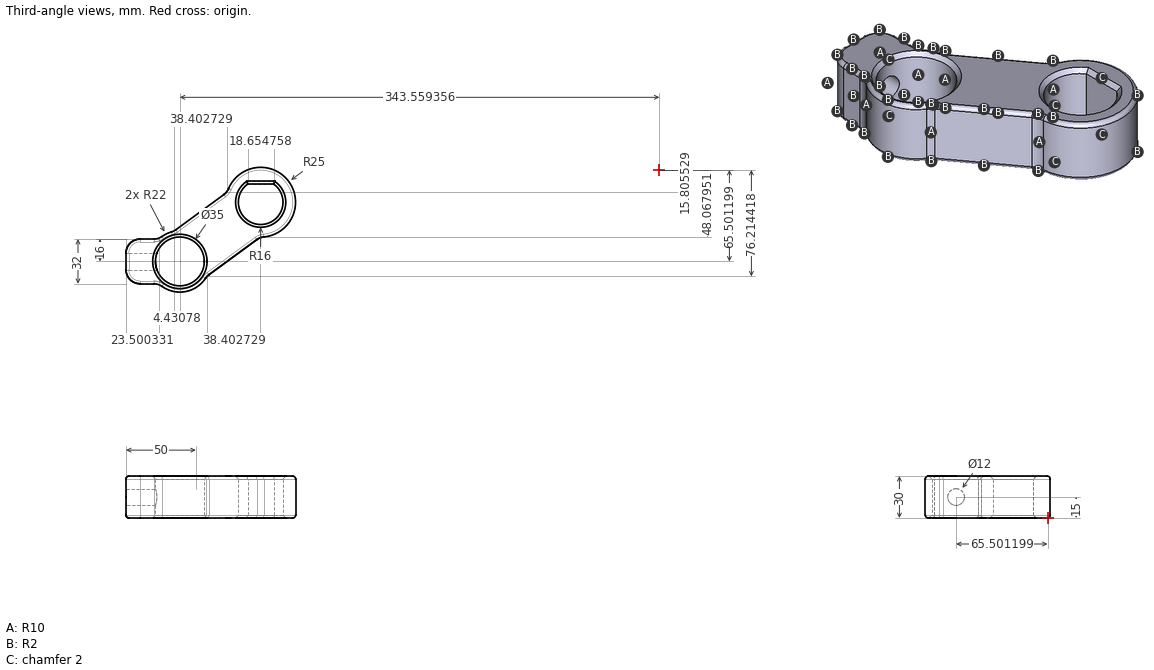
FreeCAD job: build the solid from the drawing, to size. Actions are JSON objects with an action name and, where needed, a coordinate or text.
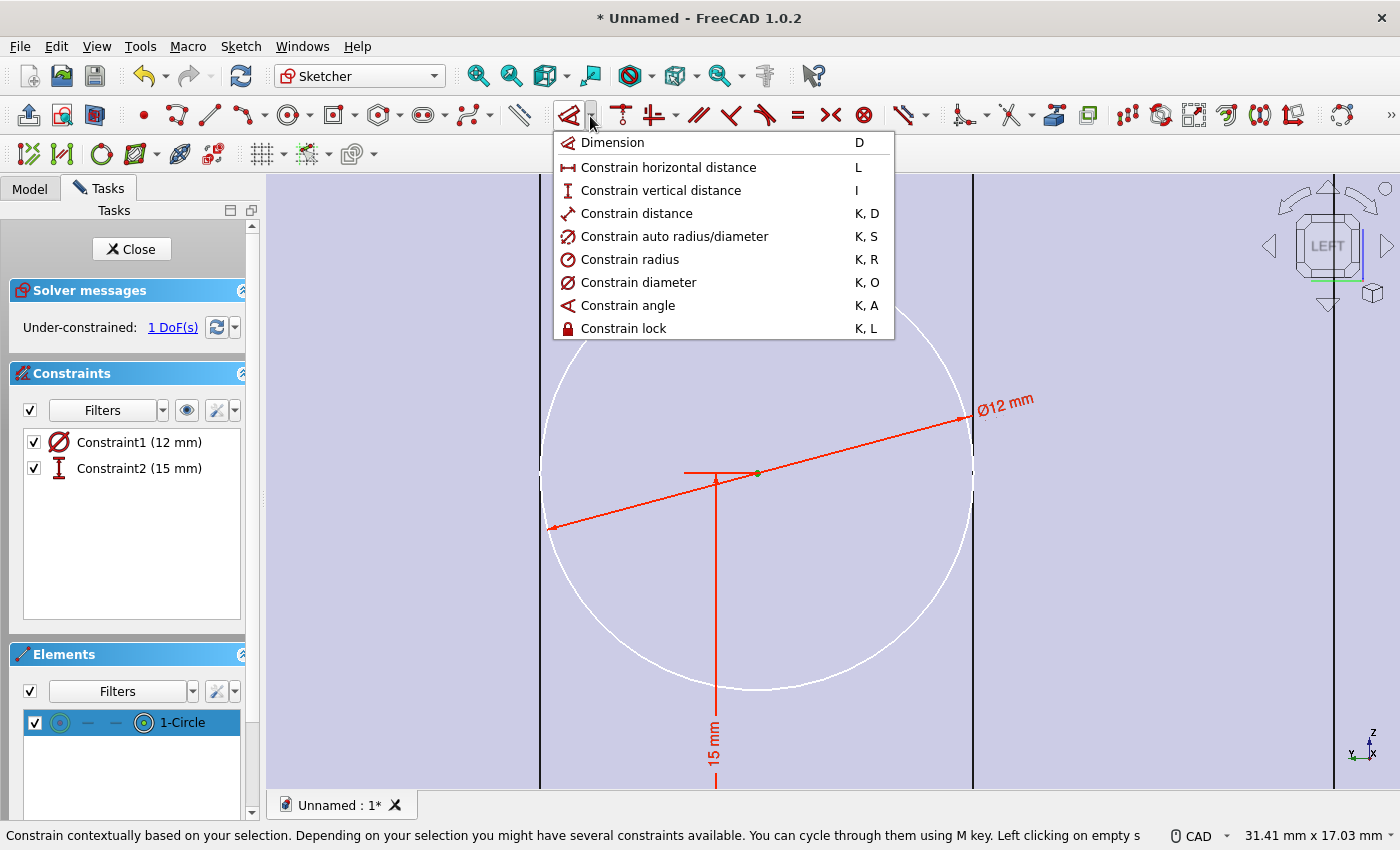
{"action": "left_click", "coordinate": [724, 168]}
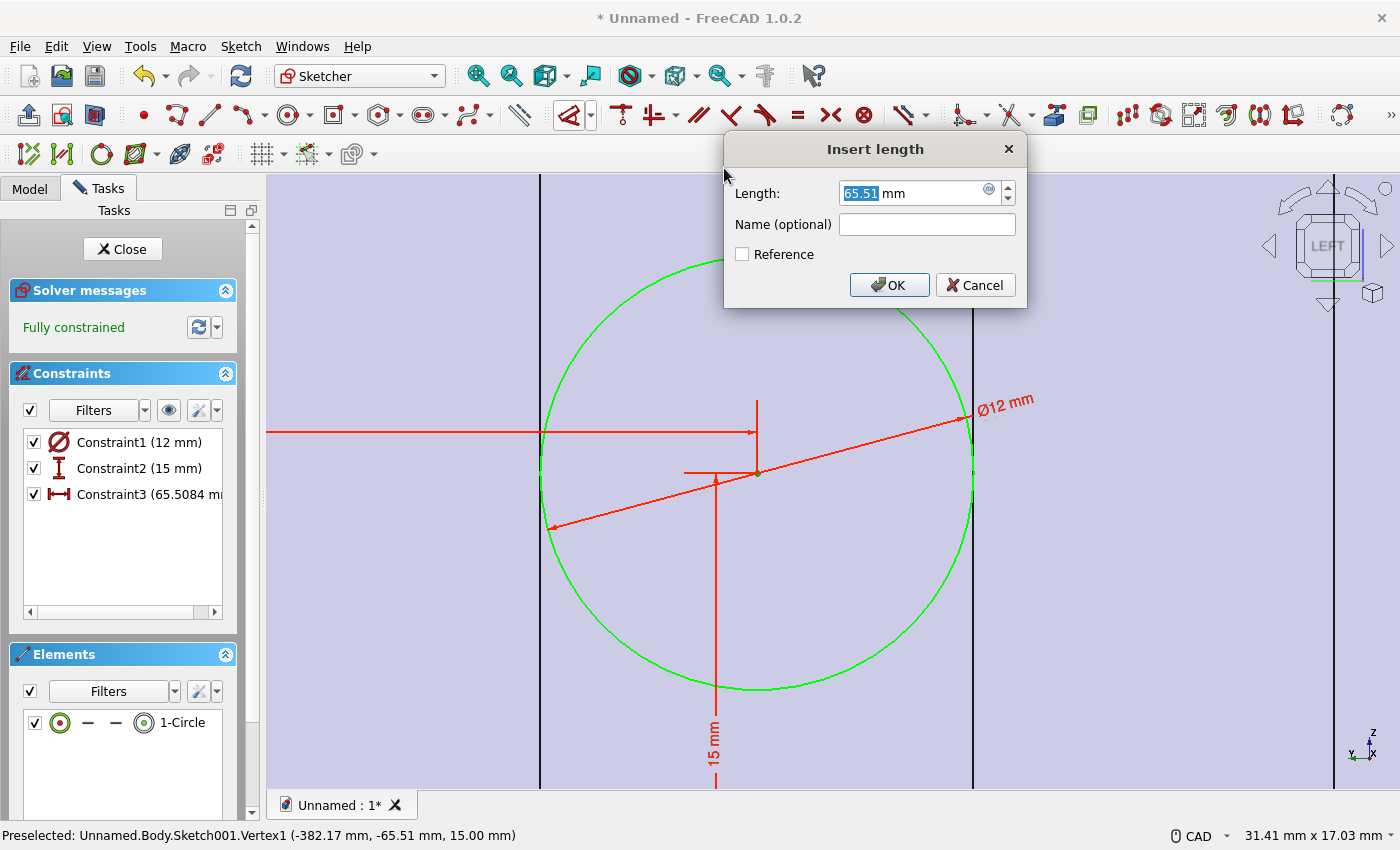
{"action": "type", "text": "65.501199"}
{"action": "key", "text": "Return"}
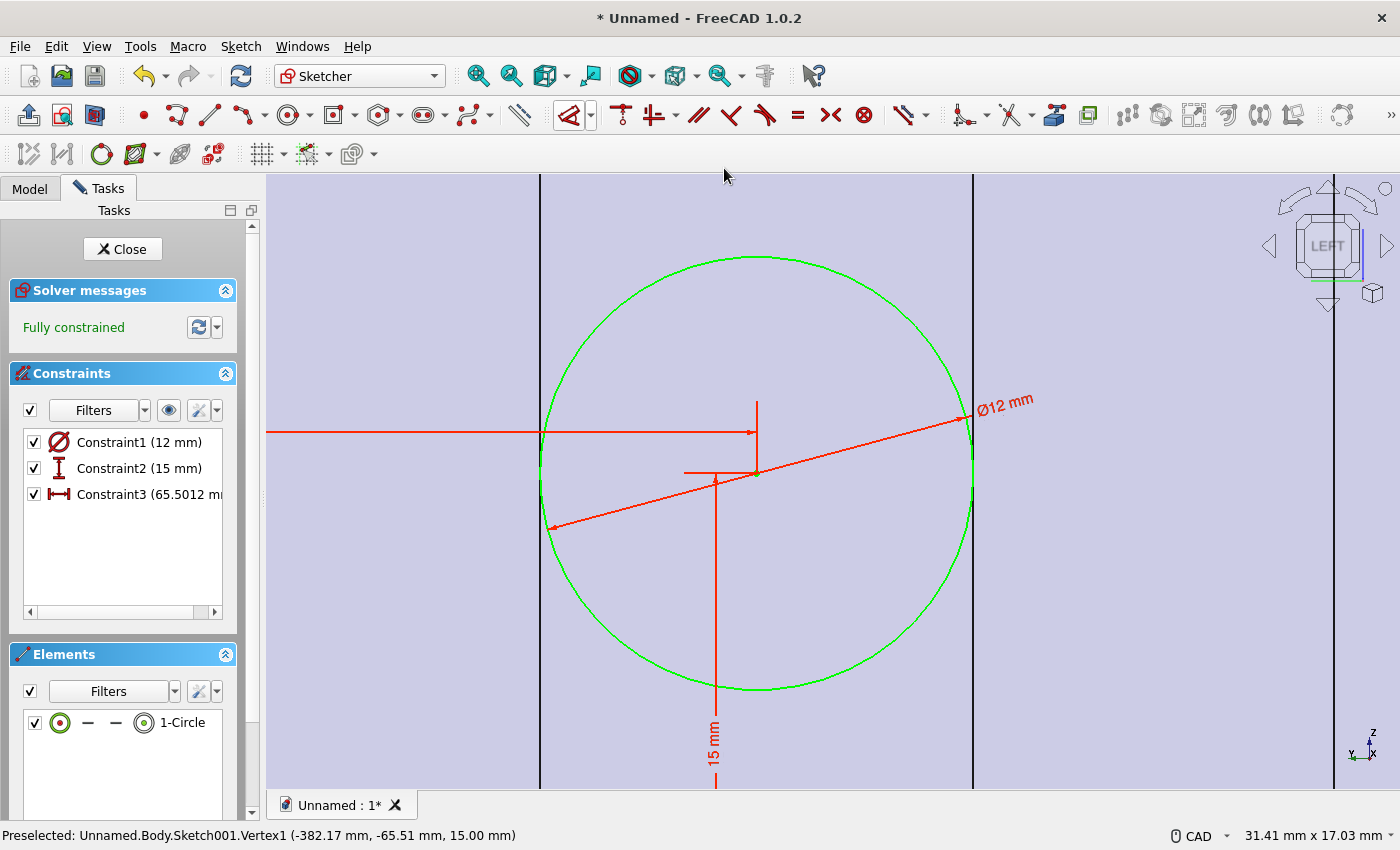
{"action": "left_click", "coordinate": [123, 249]}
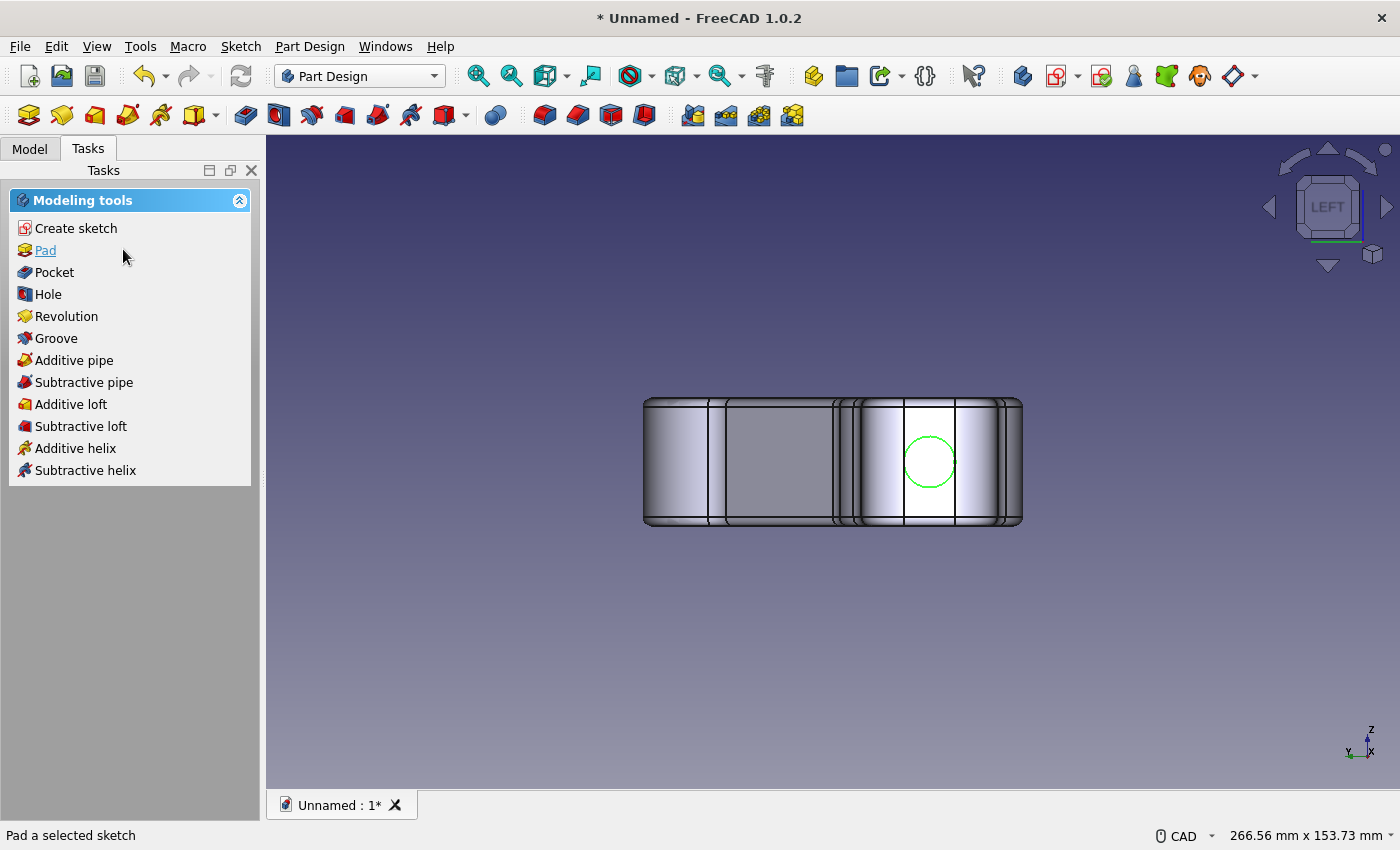
{"action": "left_click", "coordinate": [246, 116]}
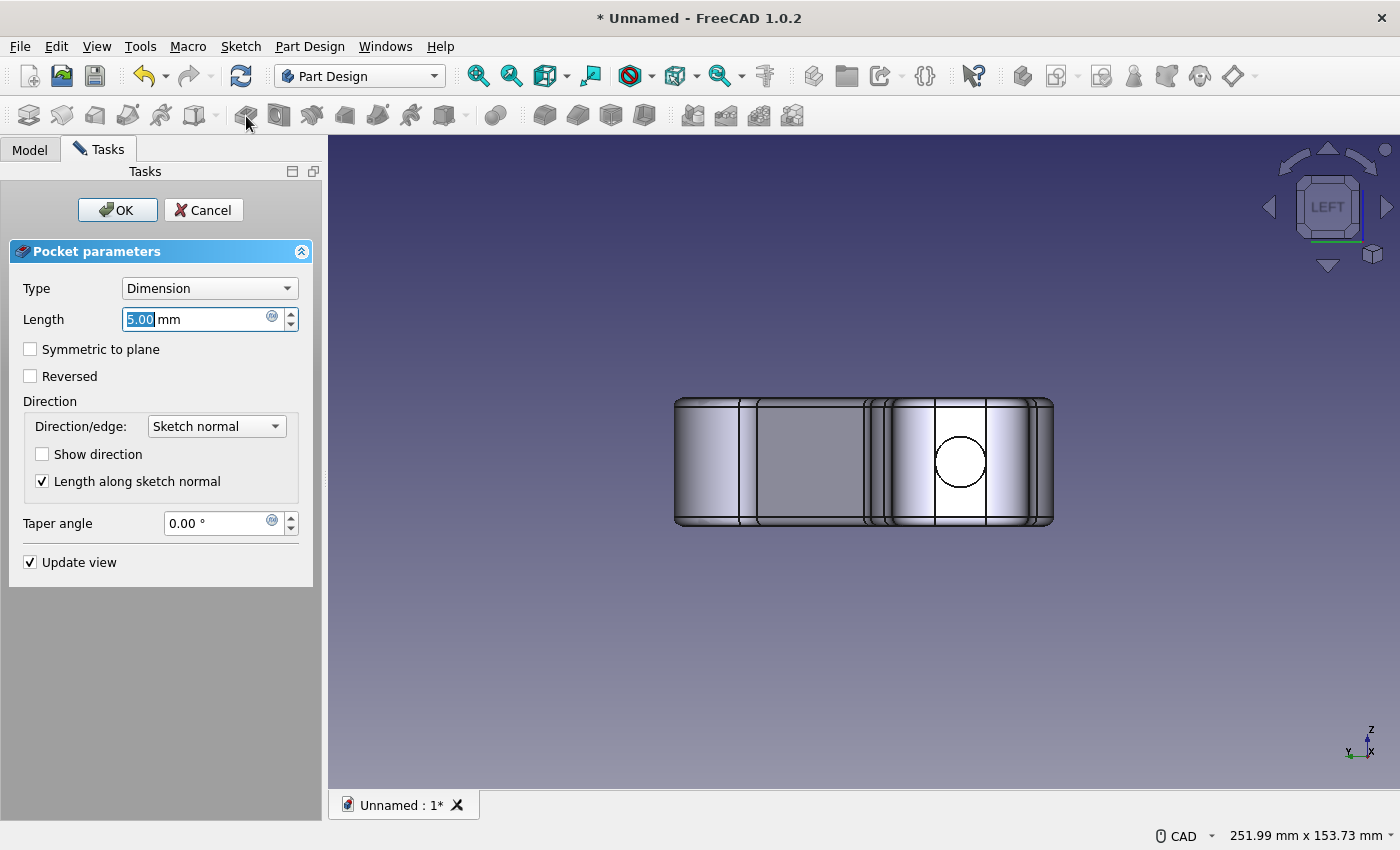
{"action": "type", "text": "50"}
{"action": "key", "text": "Tab"}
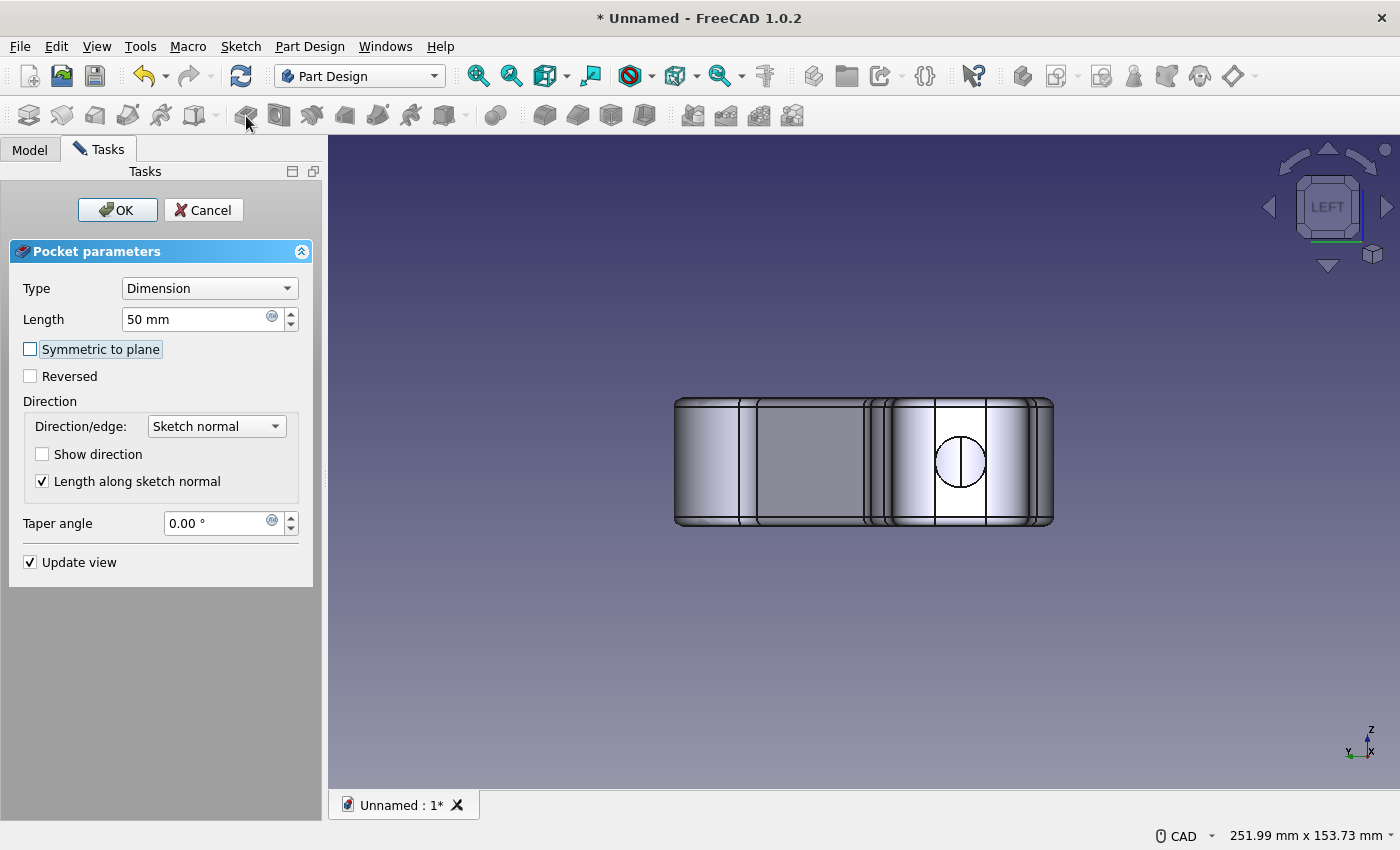
{"action": "left_click", "coordinate": [118, 210]}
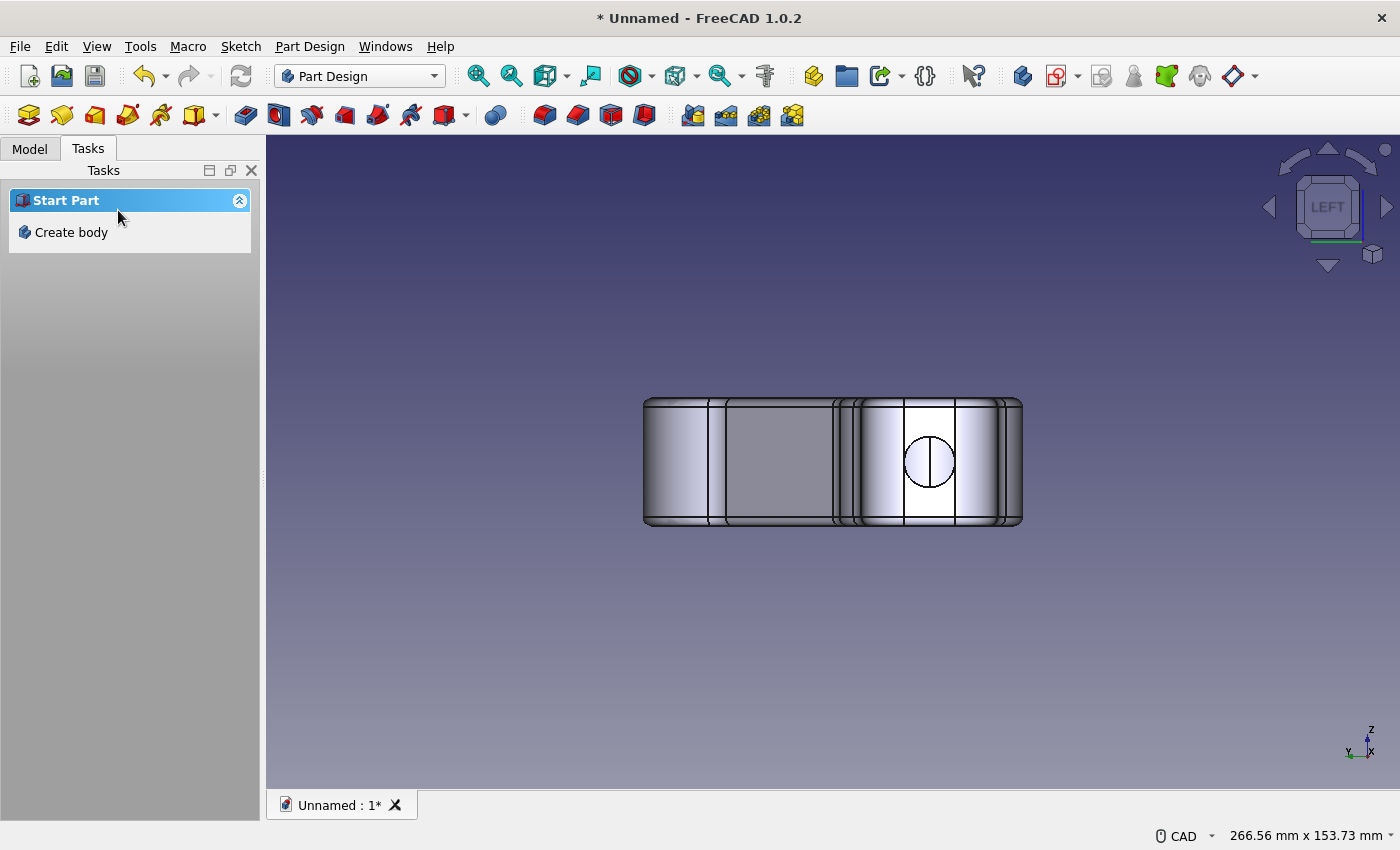
{"action": "key", "text": "0"}